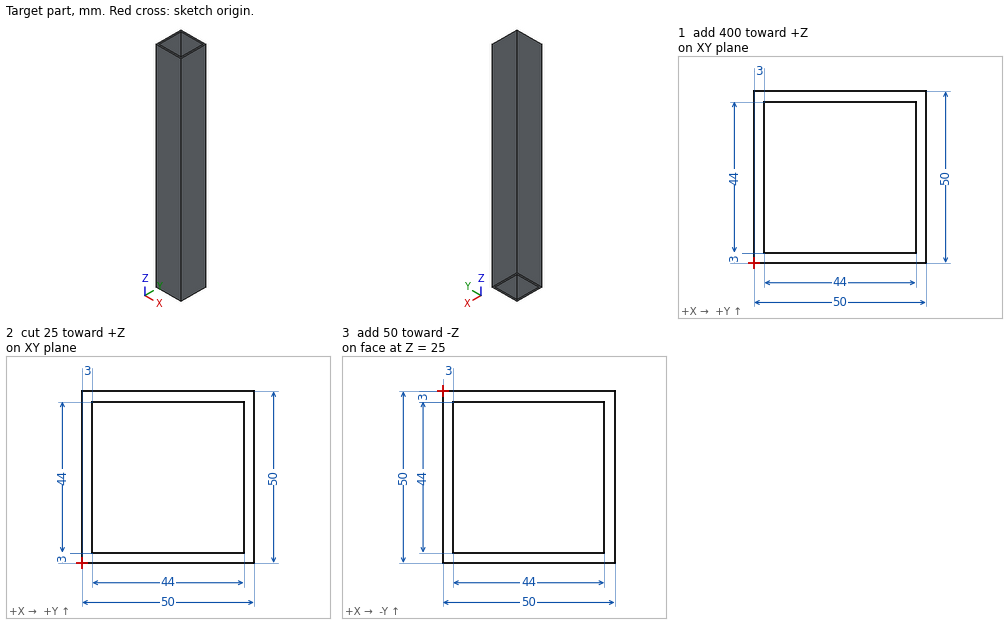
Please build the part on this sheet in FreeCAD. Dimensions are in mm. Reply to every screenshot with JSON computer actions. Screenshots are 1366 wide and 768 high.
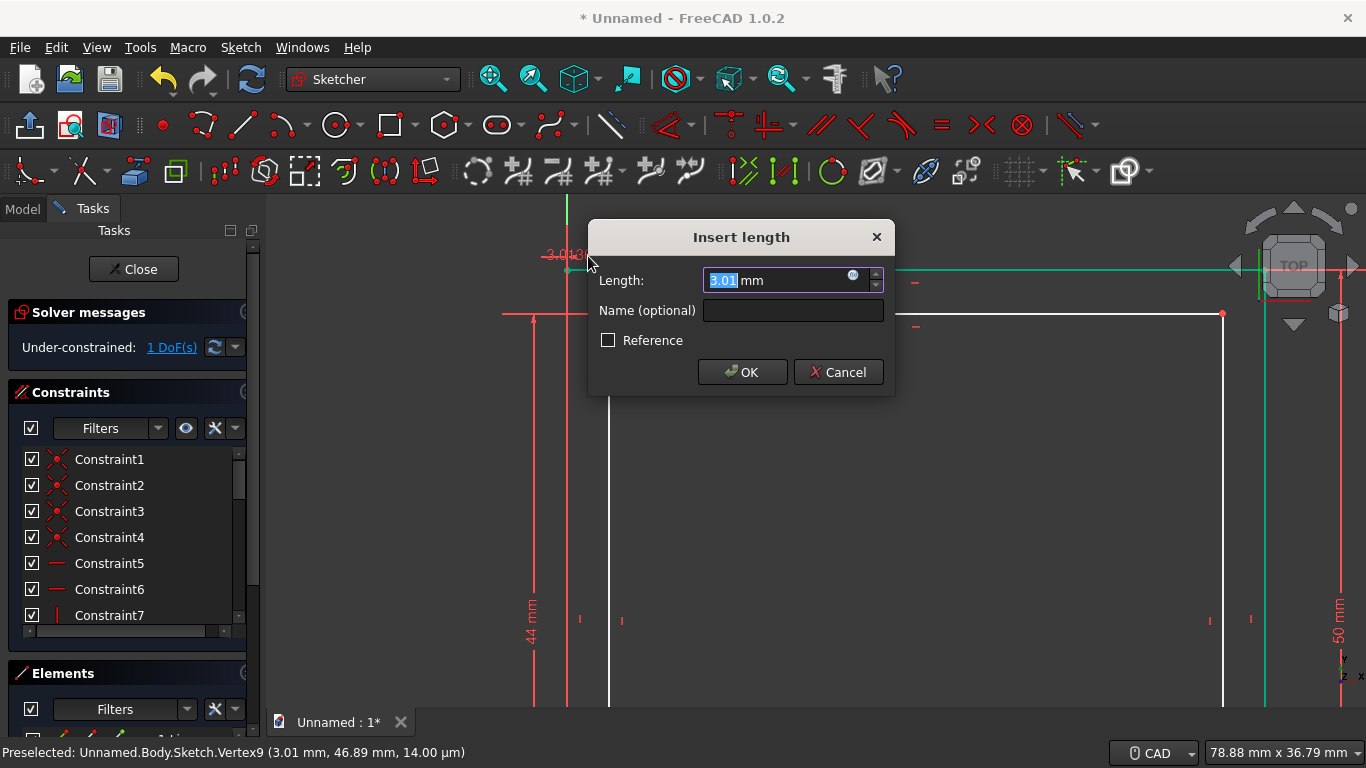
{"action": "type", "text": "3"}
{"action": "key", "text": "Return"}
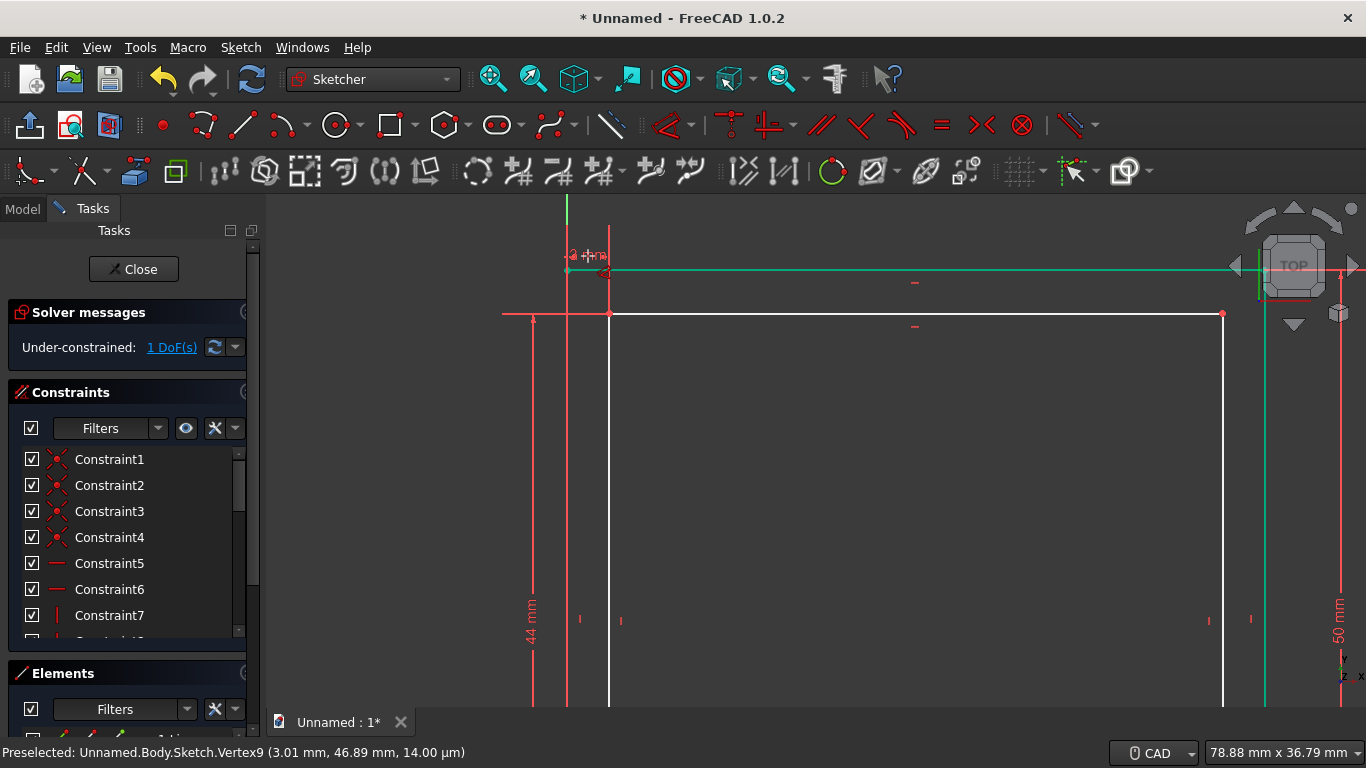
{"action": "scroll", "coordinate": [610, 313], "scroll_direction": "down", "scroll_amount": 4}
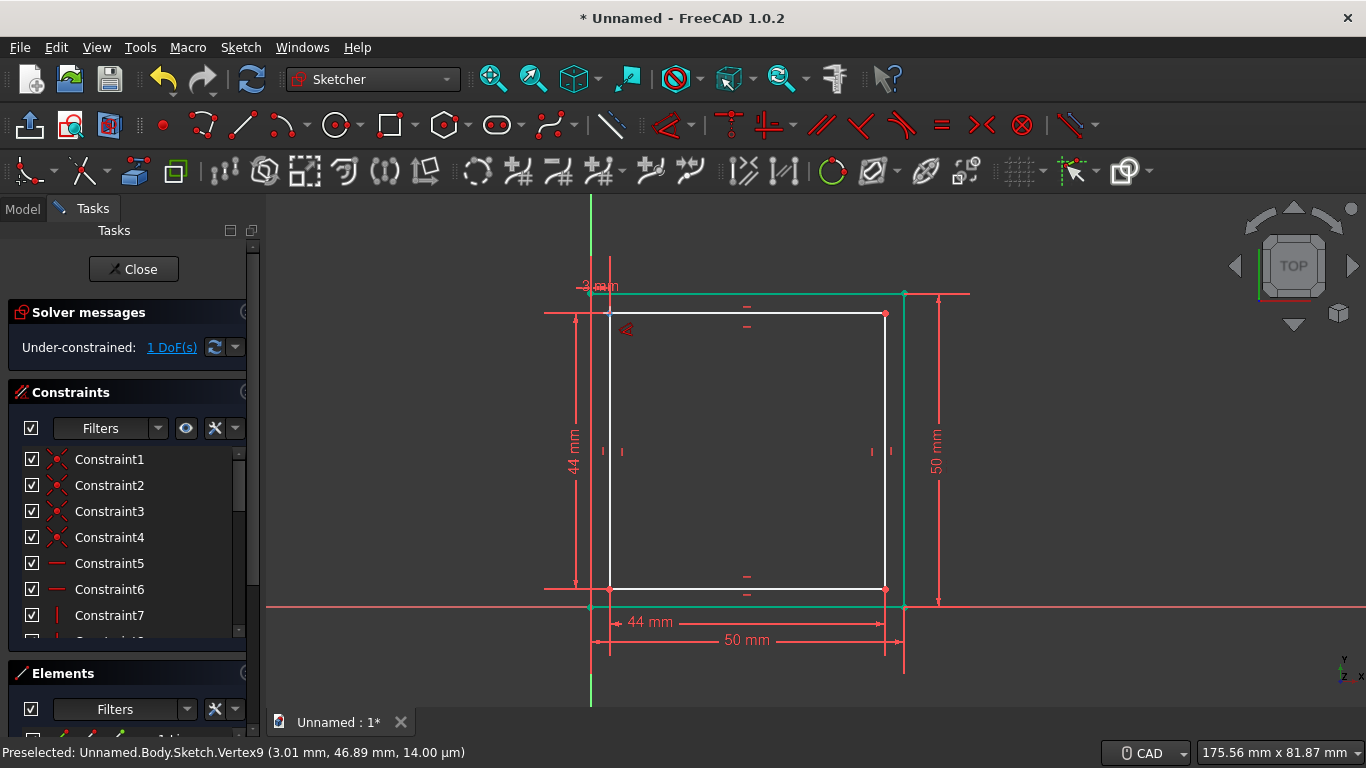
{"action": "scroll", "coordinate": [610, 589], "scroll_direction": "up", "scroll_amount": 4}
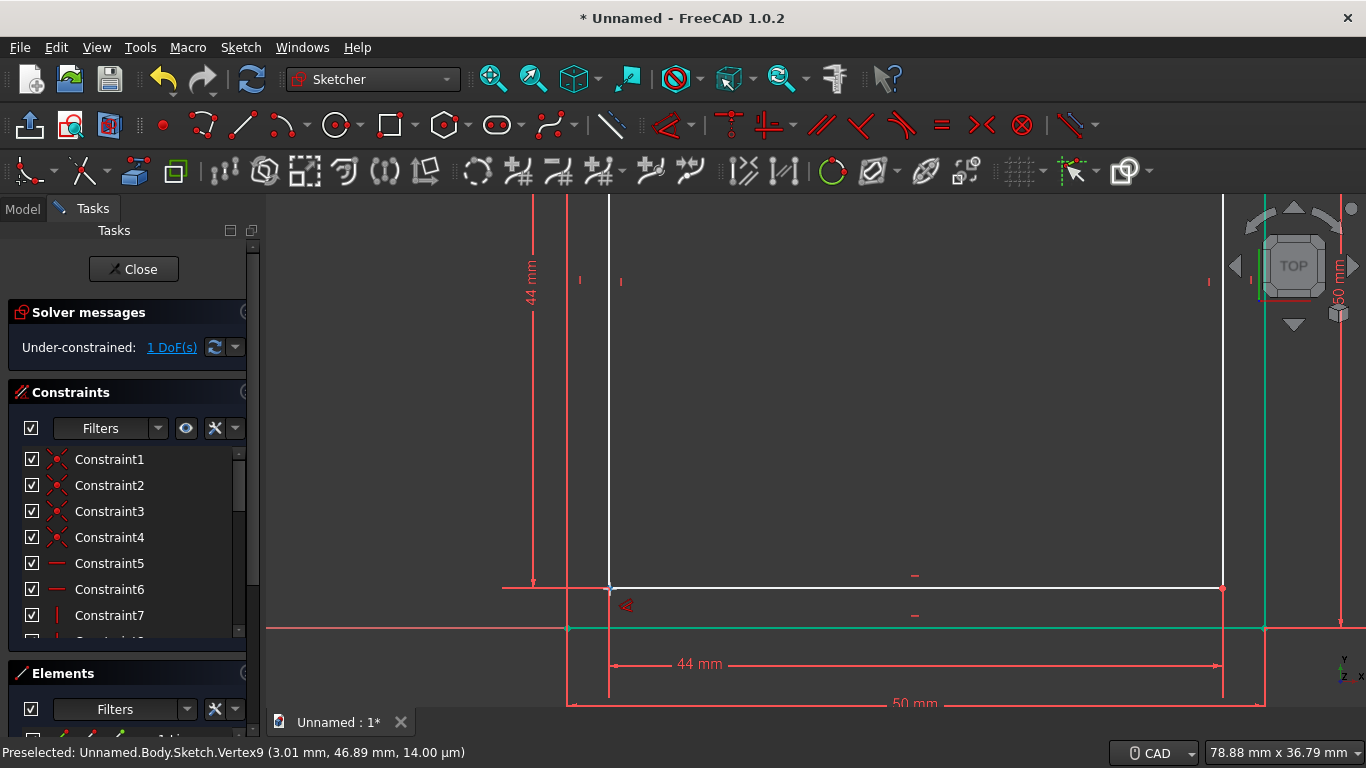
{"action": "left_click", "coordinate": [609, 588]}
{"action": "left_click", "coordinate": [533, 608]}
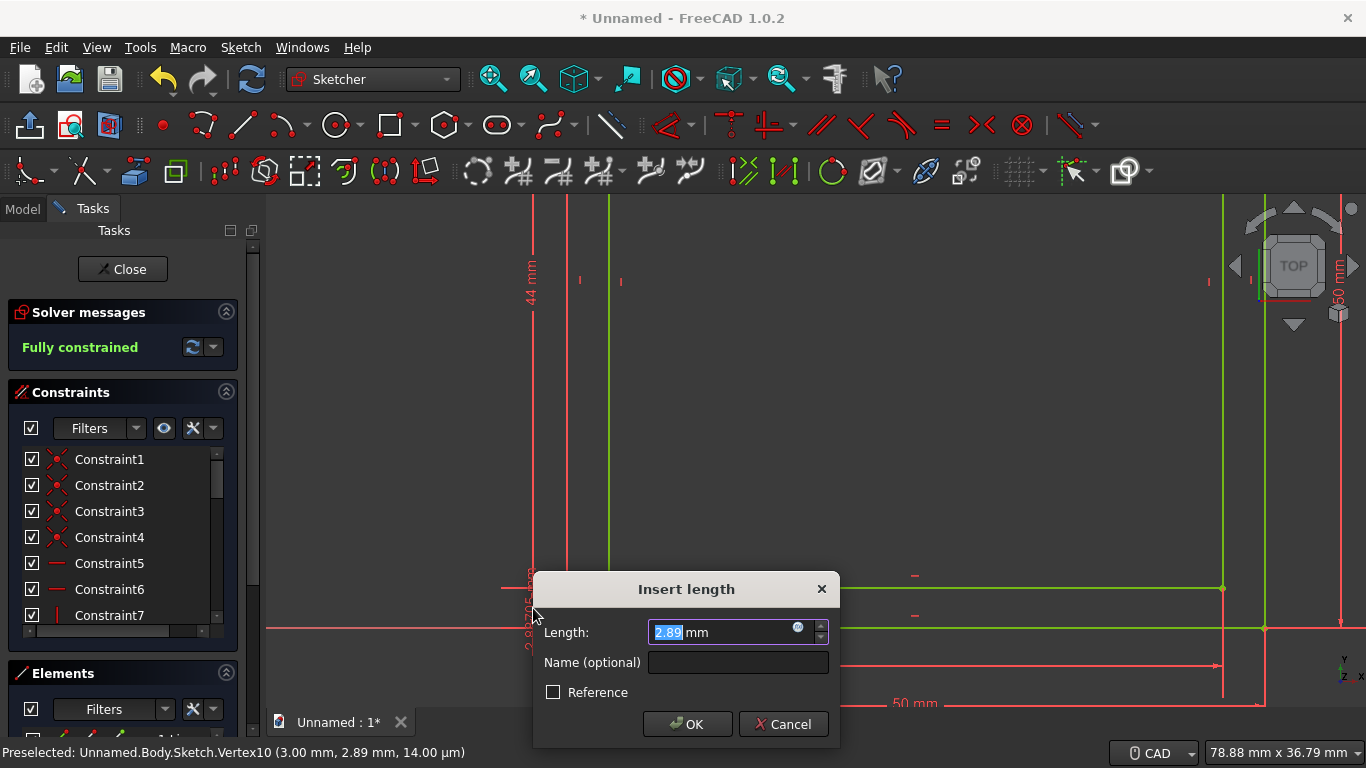
{"action": "type", "text": "3"}
{"action": "key", "text": "Return"}
{"action": "key", "text": "Escape"}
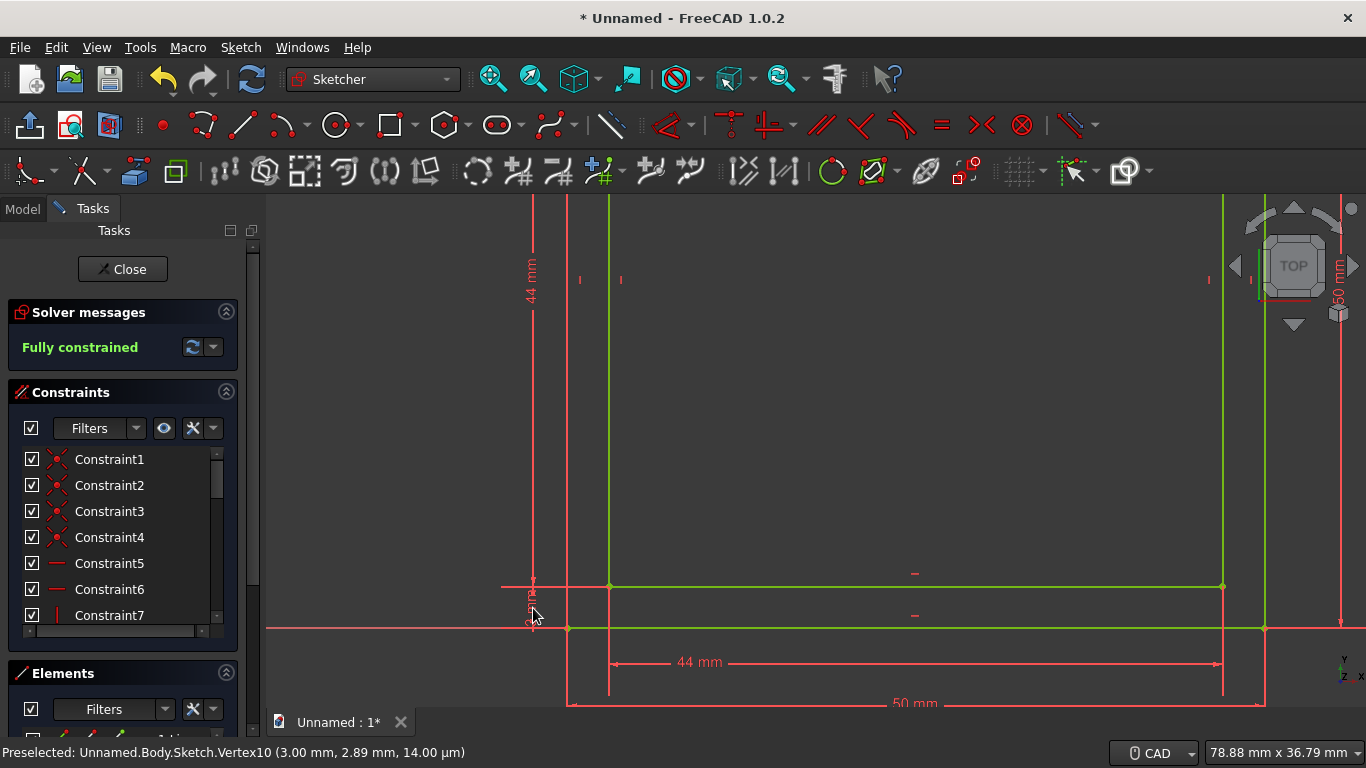
{"action": "left_click", "coordinate": [123, 269]}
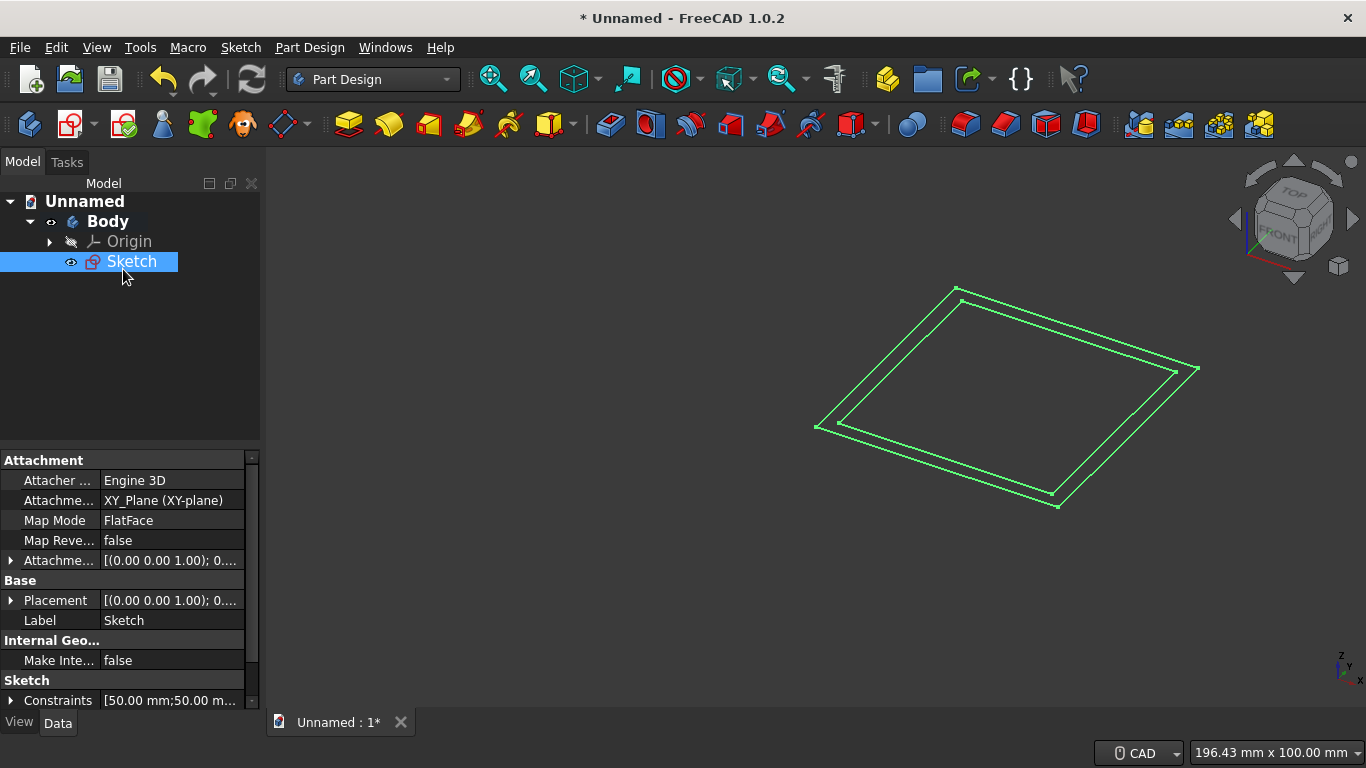
{"action": "left_click", "coordinate": [350, 124]}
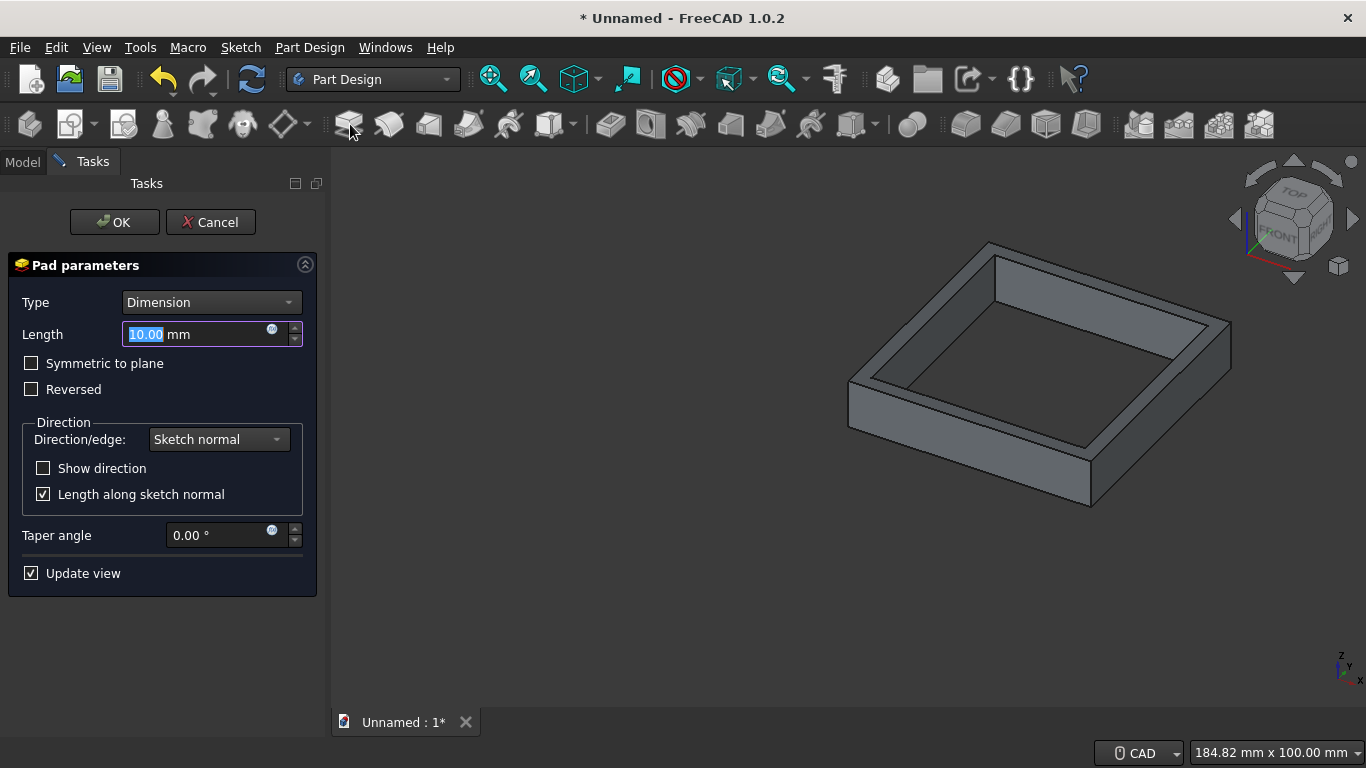
{"action": "type", "text": "400"}
{"action": "key", "text": "Tab"}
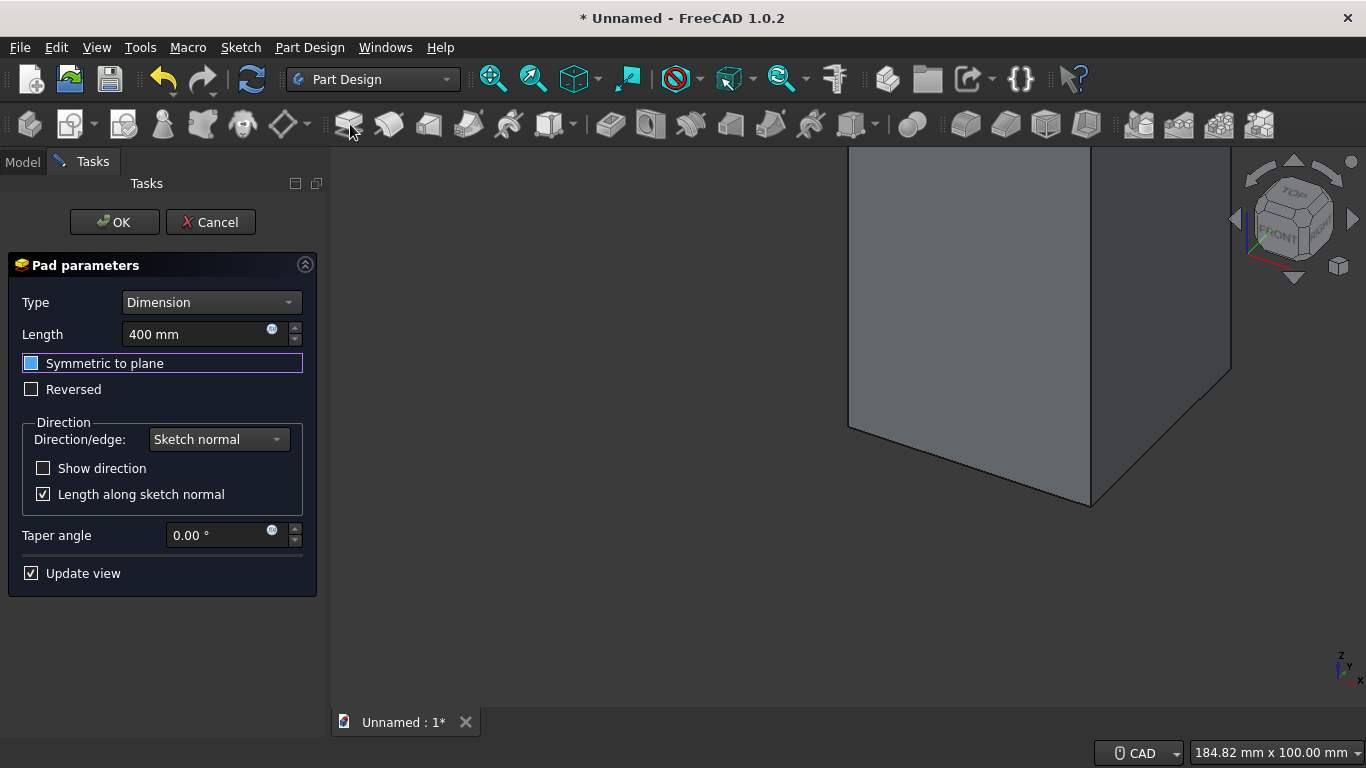
{"action": "left_click", "coordinate": [115, 222]}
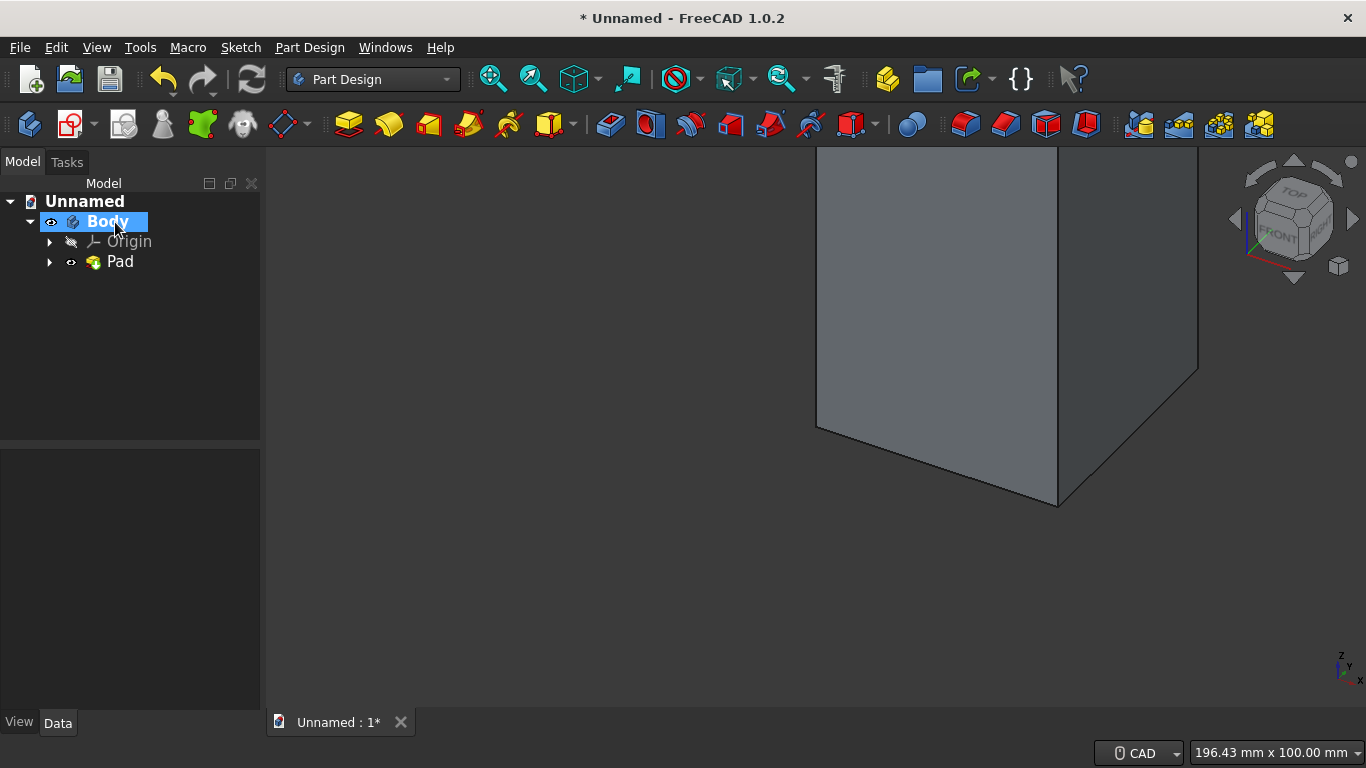
{"action": "left_click", "coordinate": [494, 80]}